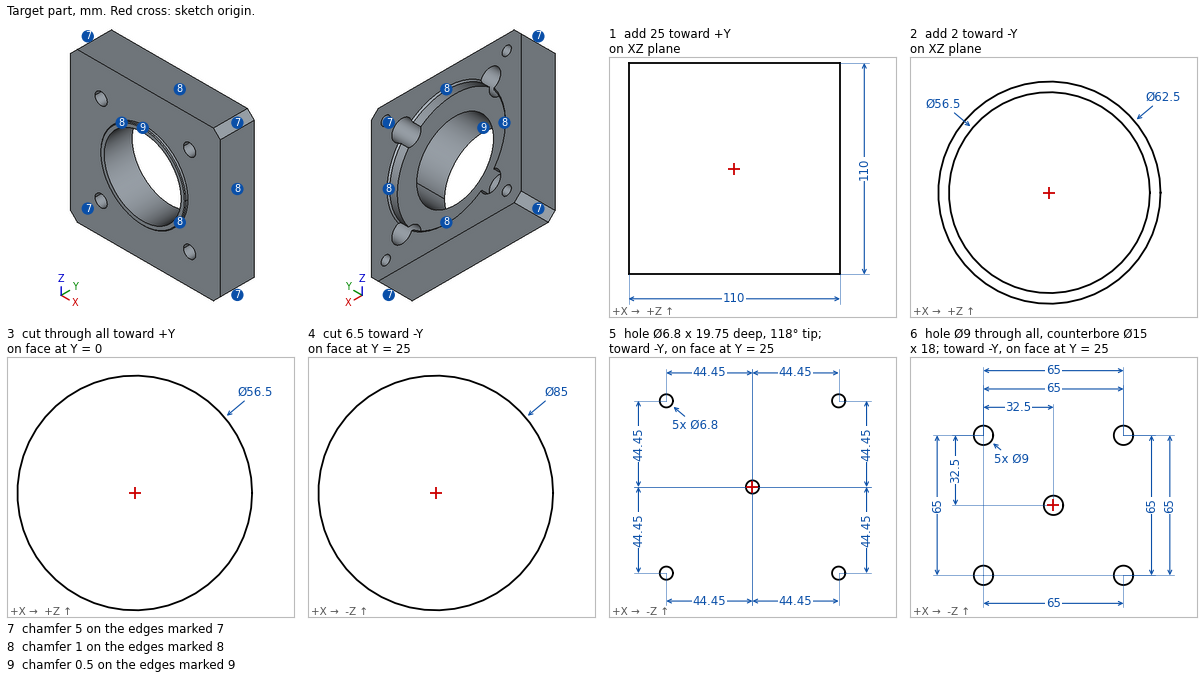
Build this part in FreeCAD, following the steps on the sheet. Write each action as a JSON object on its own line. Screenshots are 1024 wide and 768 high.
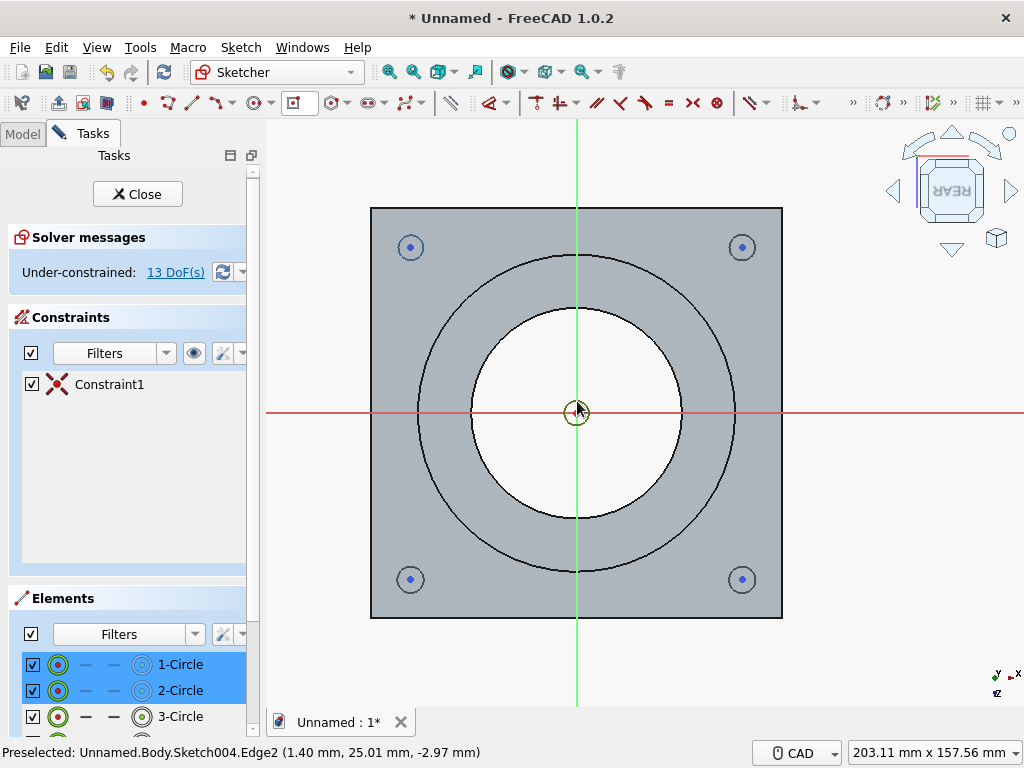
{"action": "left_click", "coordinate": [751, 239]}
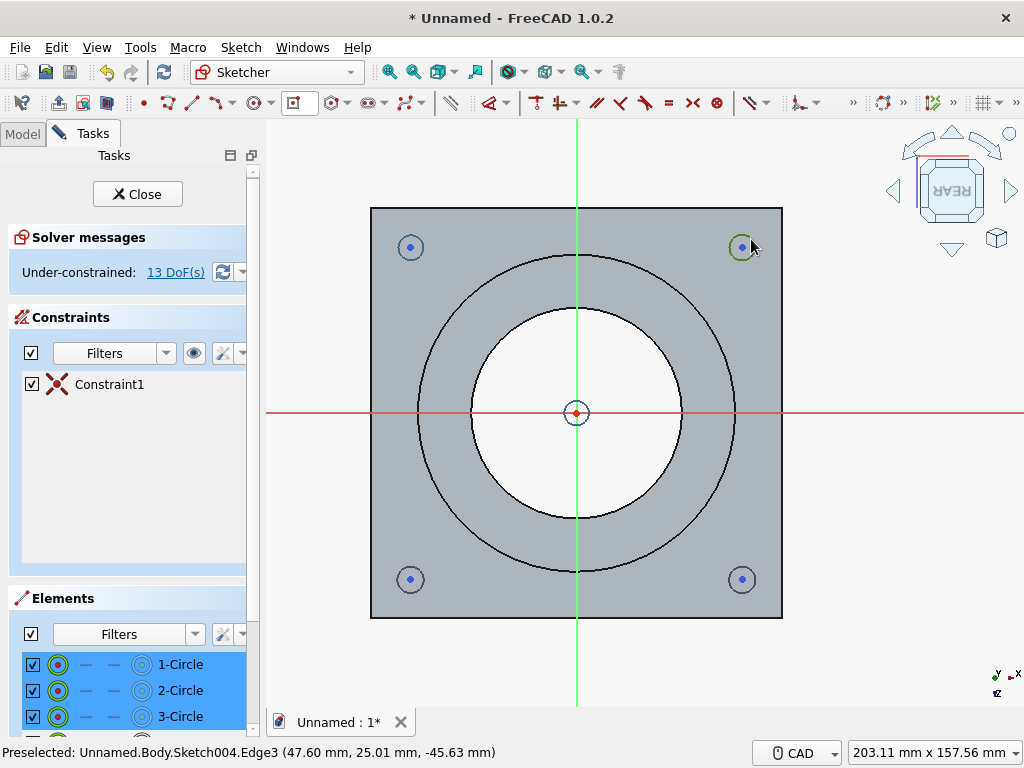
{"action": "left_click", "coordinate": [420, 571]}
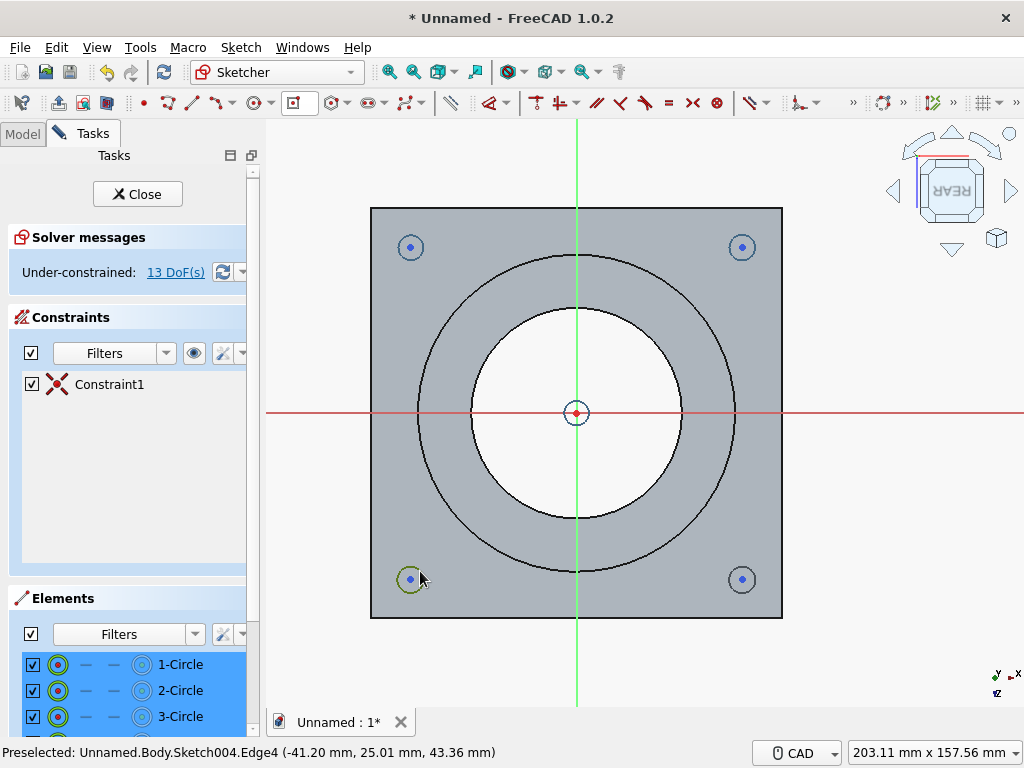
{"action": "left_click", "coordinate": [752, 571]}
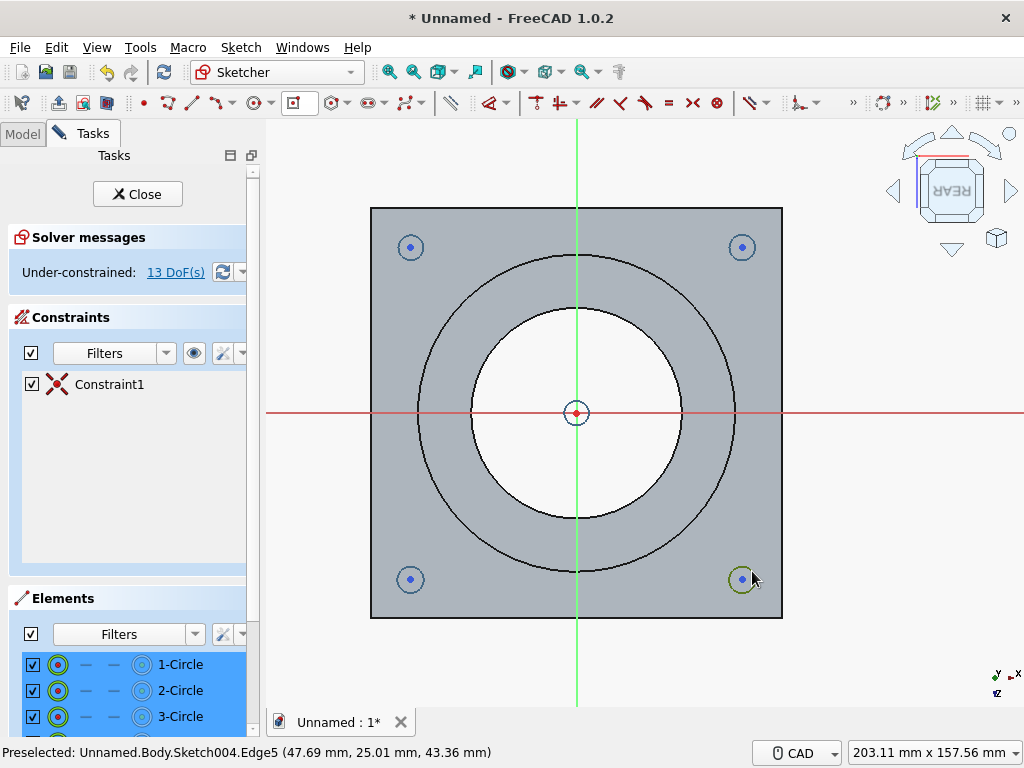
{"action": "left_click", "coordinate": [670, 104]}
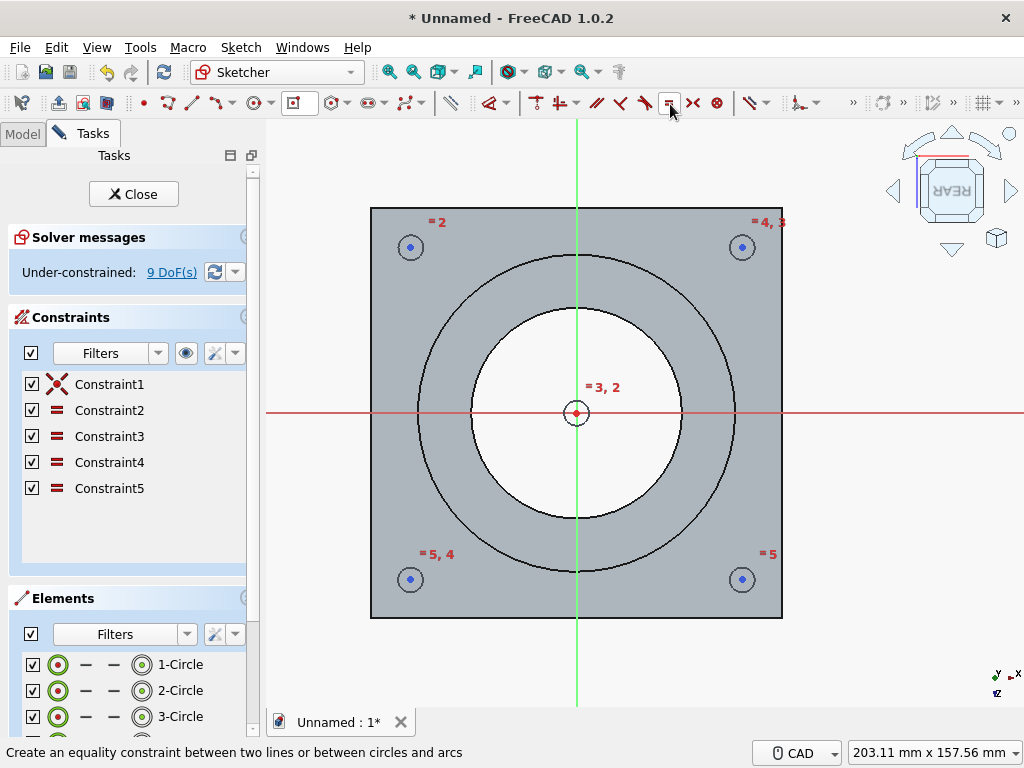
{"action": "left_click", "coordinate": [490, 104]}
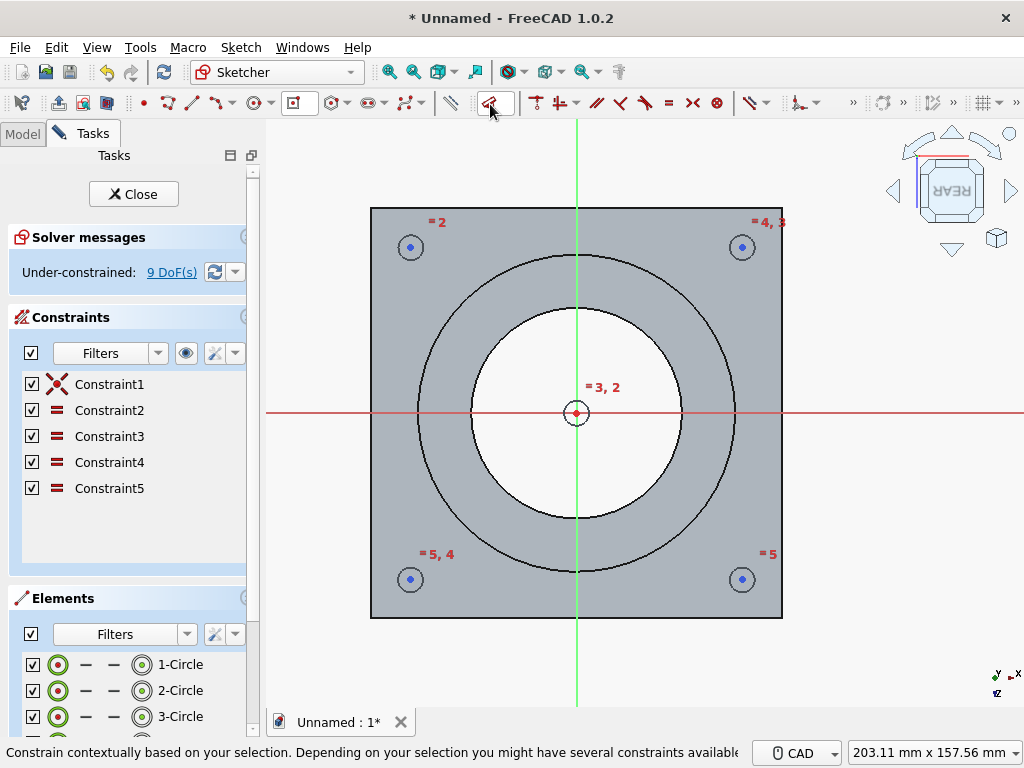
{"action": "scroll", "coordinate": [420, 239], "scroll_direction": "up", "scroll_amount": 3}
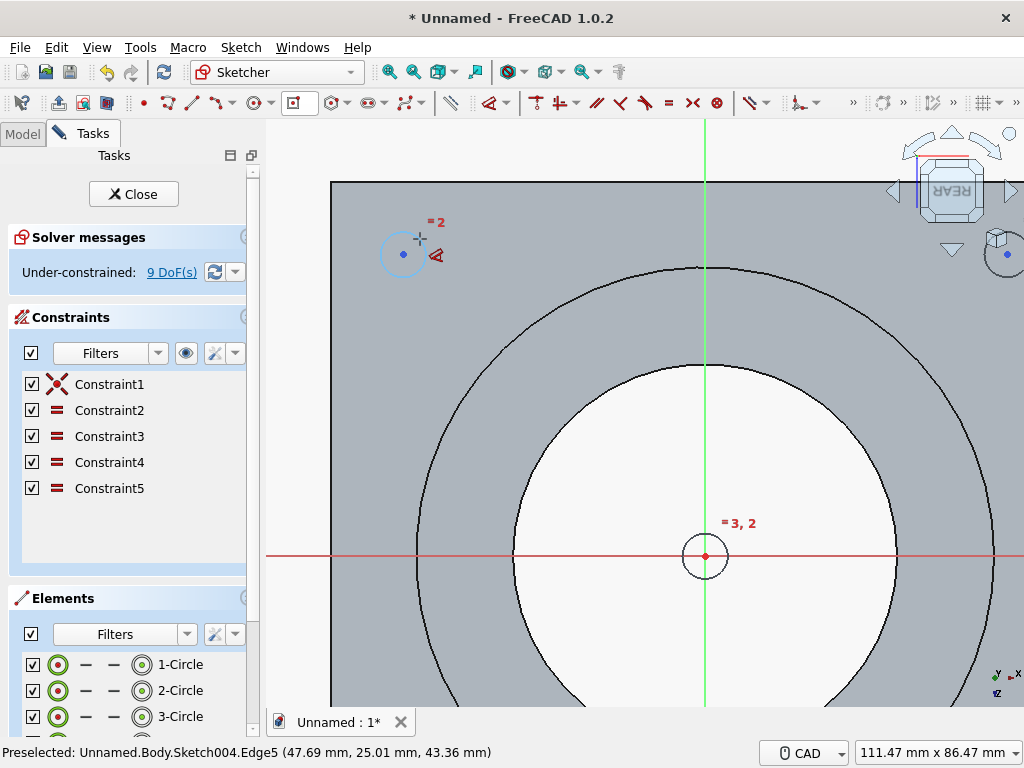
{"action": "left_click", "coordinate": [419, 239]}
{"action": "left_click", "coordinate": [442, 216]}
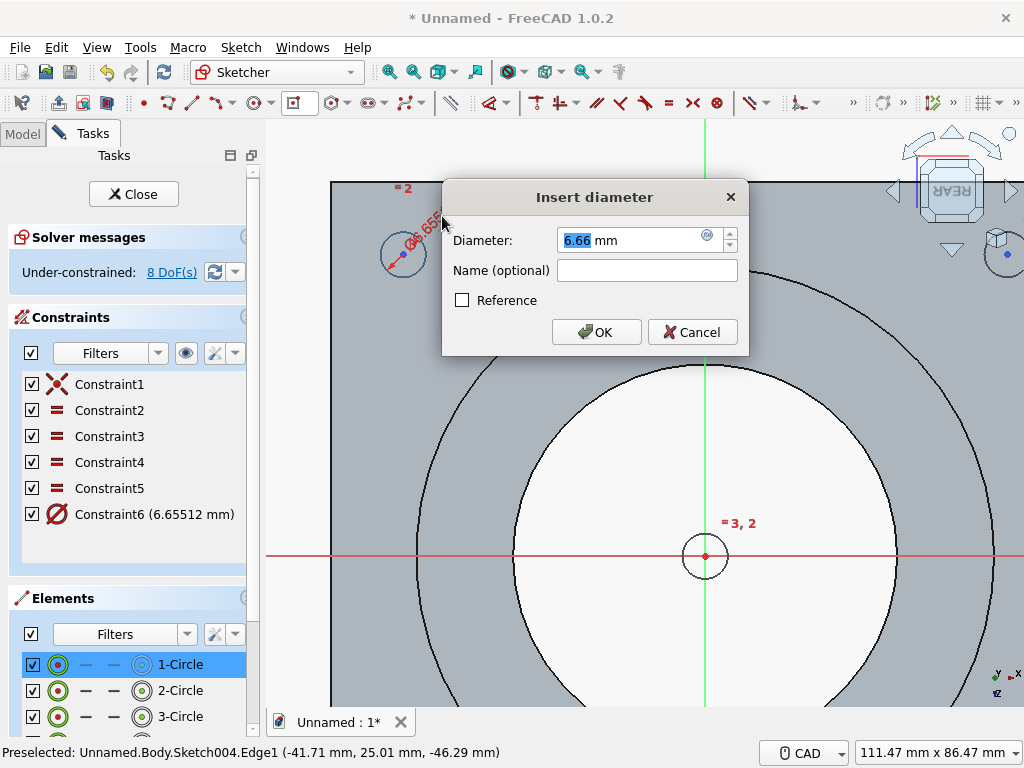
{"action": "type", "text": "6.8"}
{"action": "key", "text": "Return"}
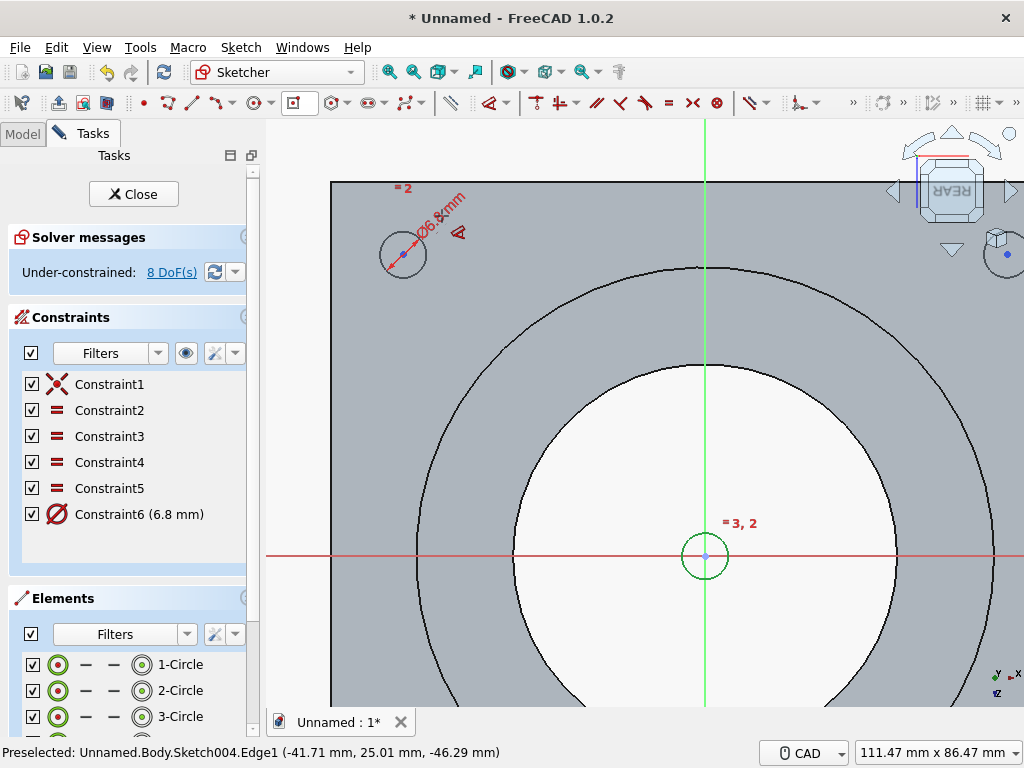
{"action": "left_click", "coordinate": [403, 255]}
{"action": "left_click", "coordinate": [554, 221]}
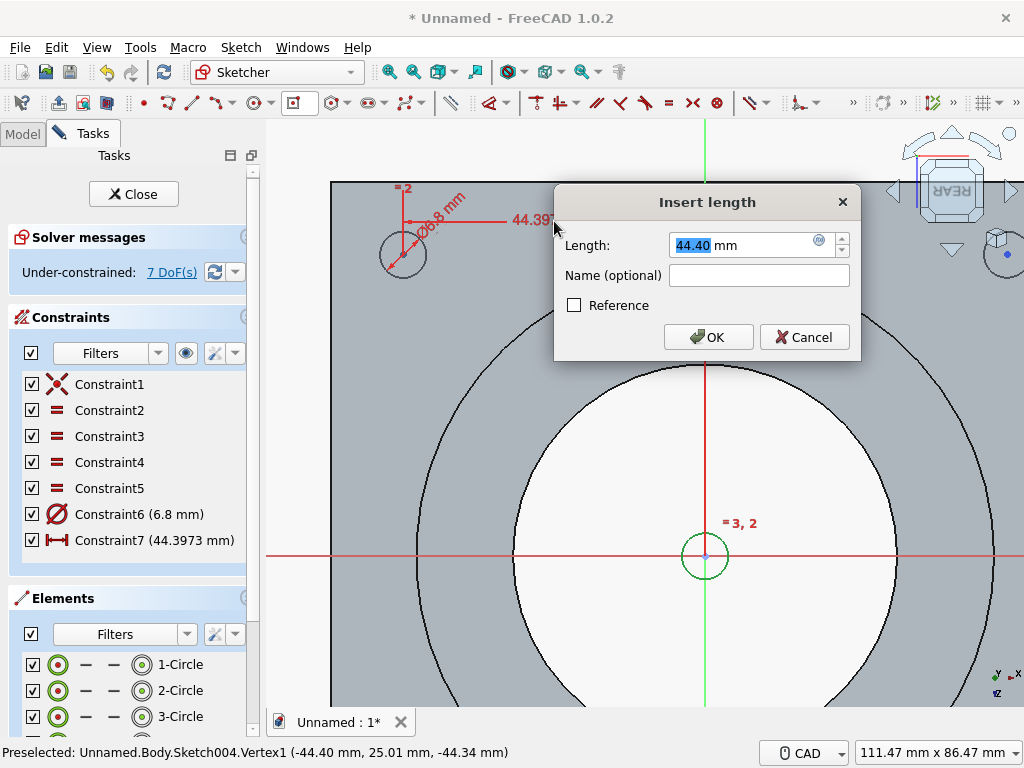
{"action": "type", "text": "44.45"}
{"action": "key", "text": "Return"}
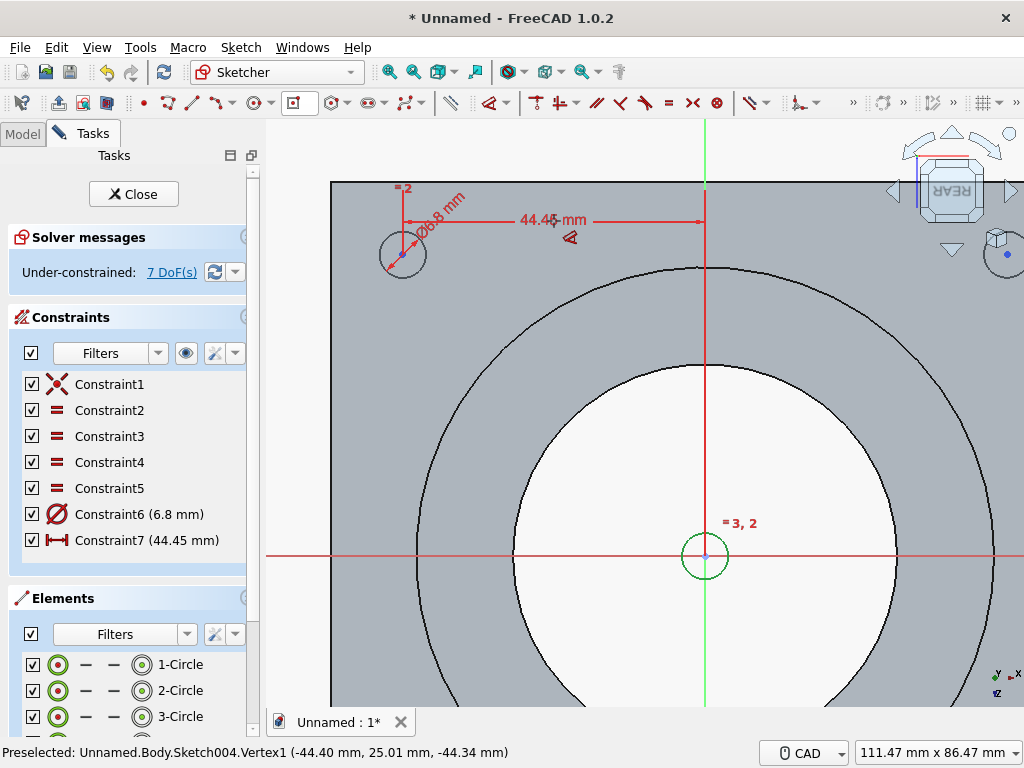
{"action": "left_click", "coordinate": [403, 255]}
{"action": "left_click", "coordinate": [369, 406]}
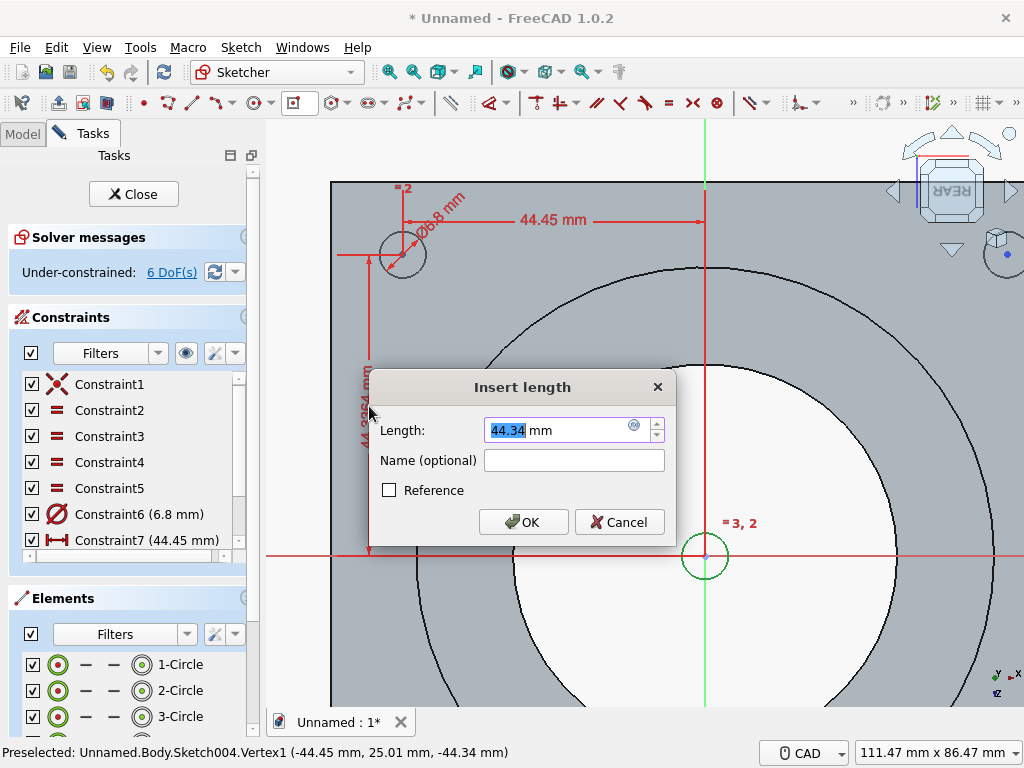
{"action": "type", "text": "44.45"}
{"action": "key", "text": "Return"}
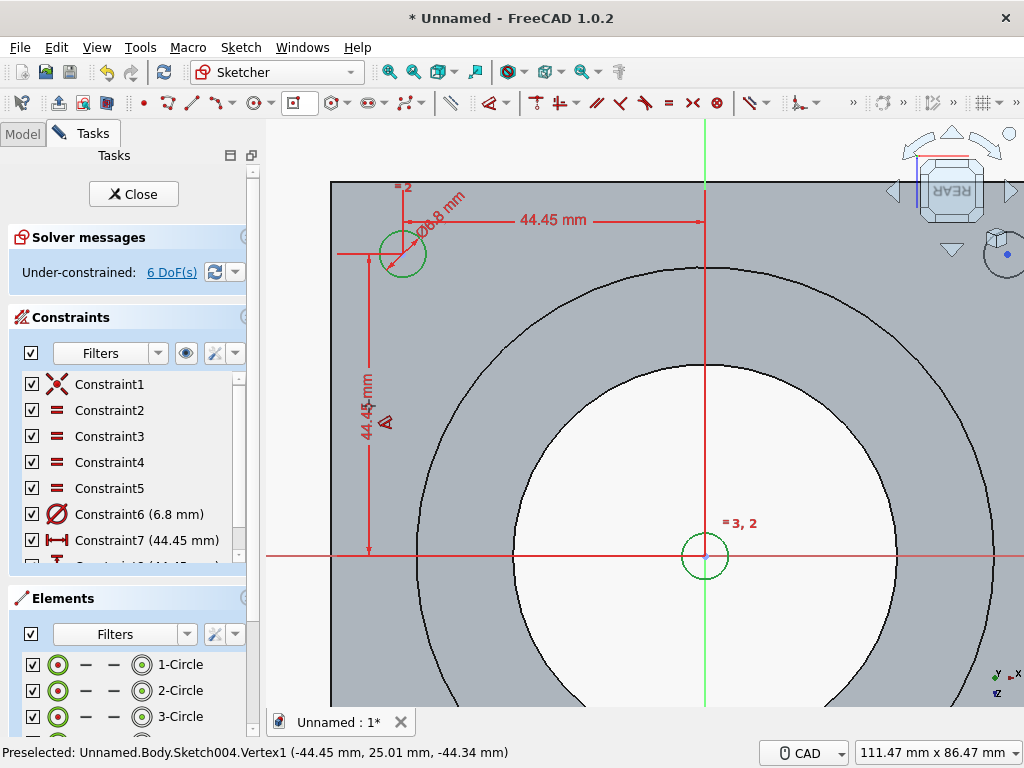
{"action": "scroll", "coordinate": [420, 239], "scroll_direction": "down", "scroll_amount": 3}